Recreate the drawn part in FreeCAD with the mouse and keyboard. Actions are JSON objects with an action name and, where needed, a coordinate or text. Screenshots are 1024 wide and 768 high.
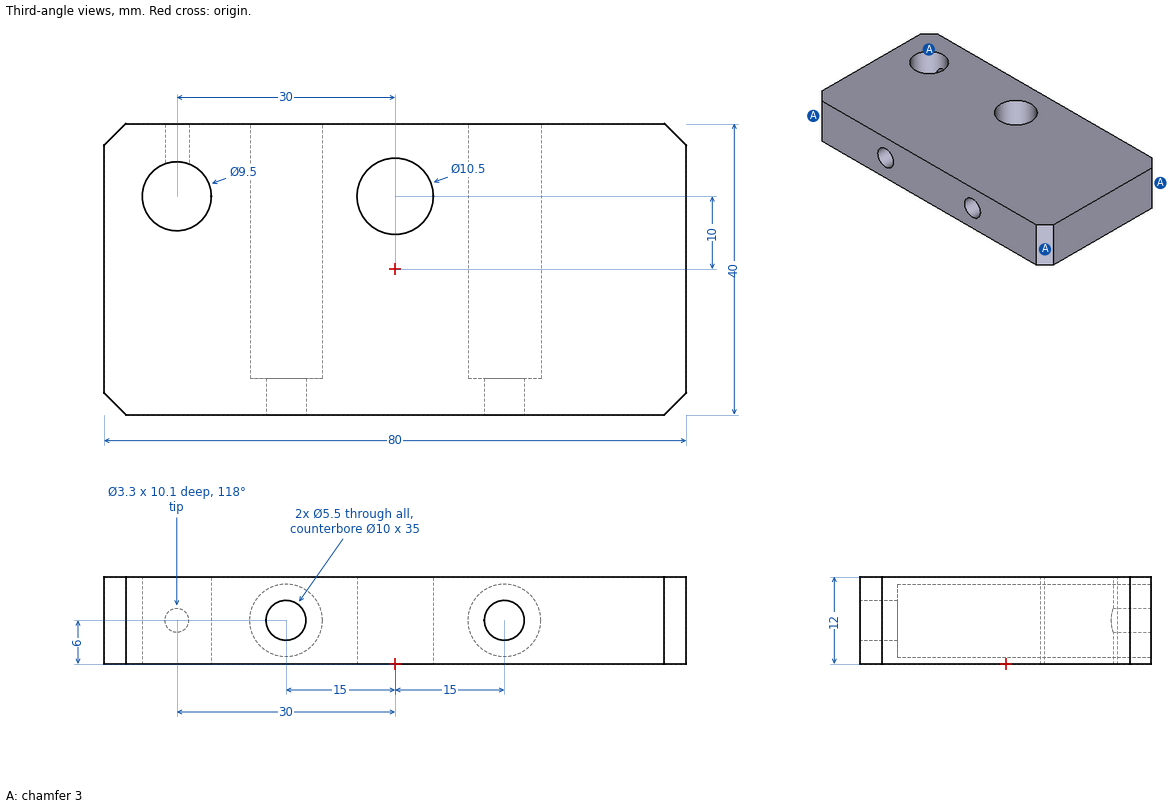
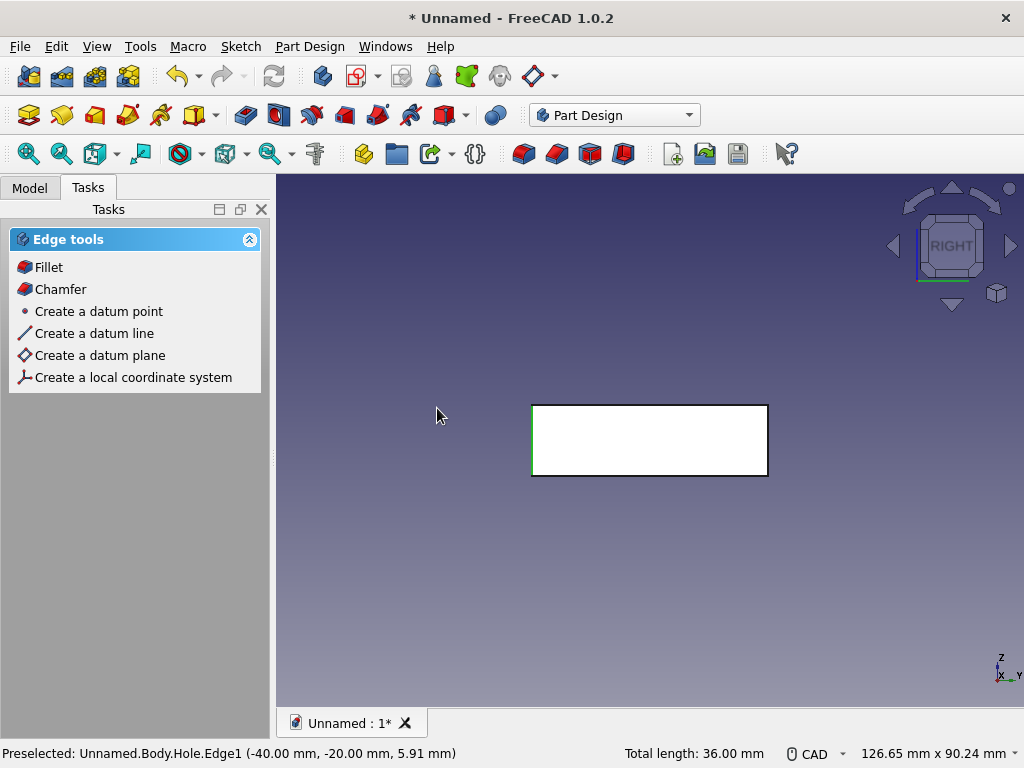
{"action": "left_click", "coordinate": [768, 439], "text": "ctrl"}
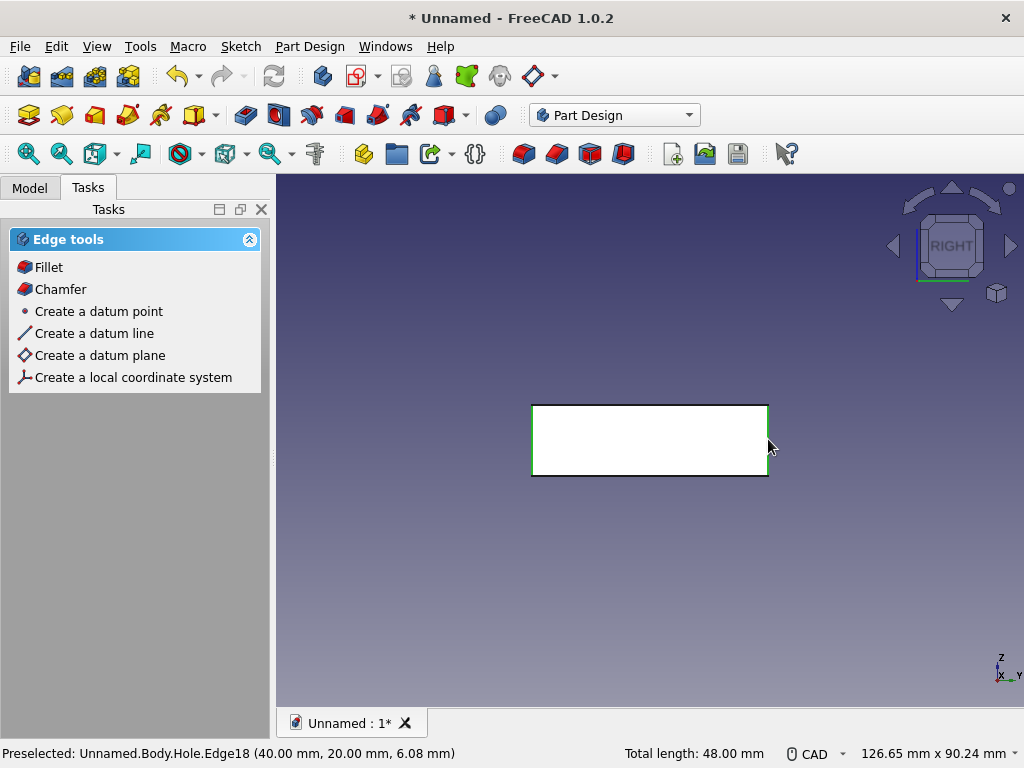
{"action": "left_click", "coordinate": [557, 154]}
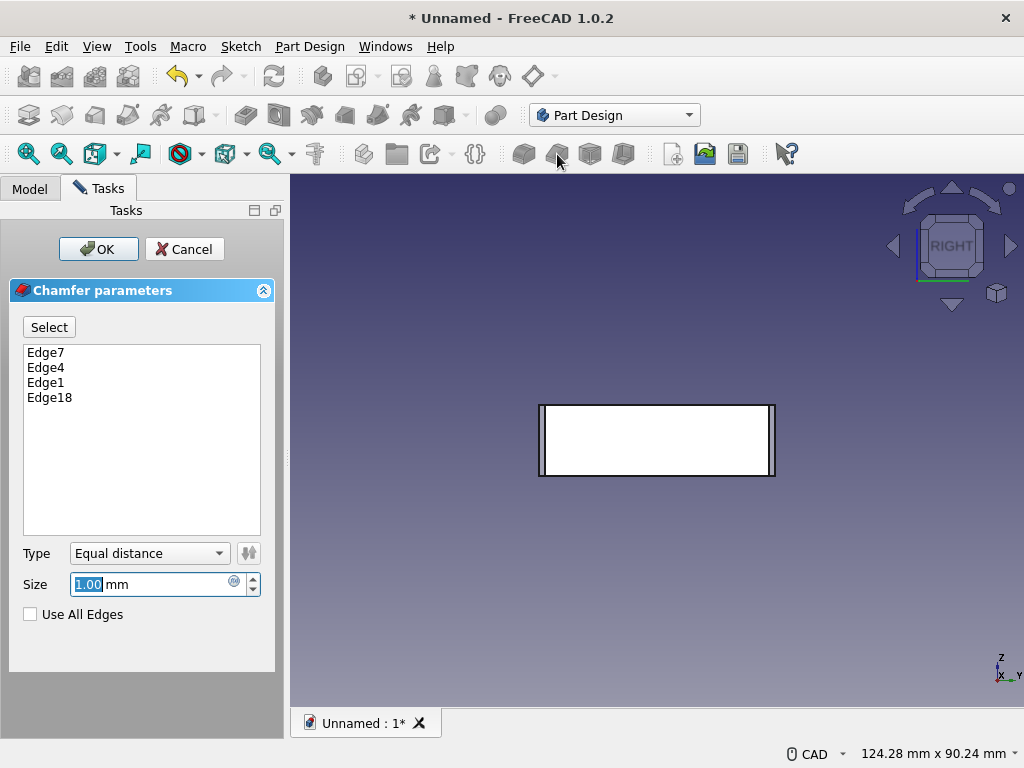
{"action": "type", "text": "3"}
{"action": "key", "text": "Tab"}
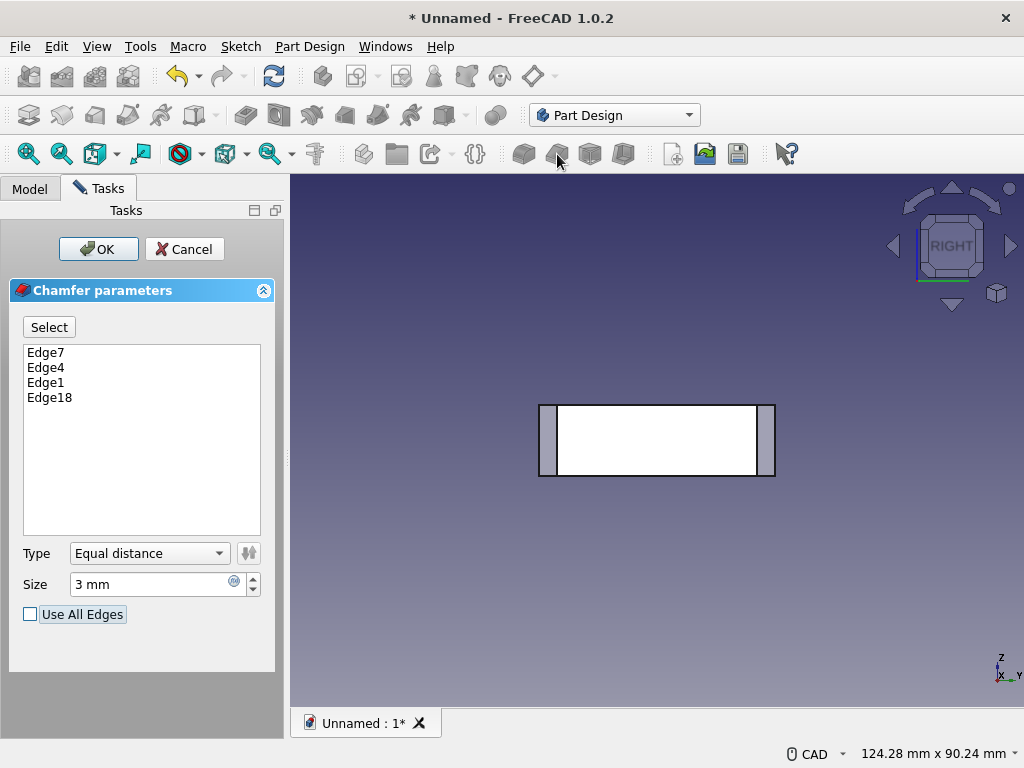
{"action": "left_click", "coordinate": [99, 249]}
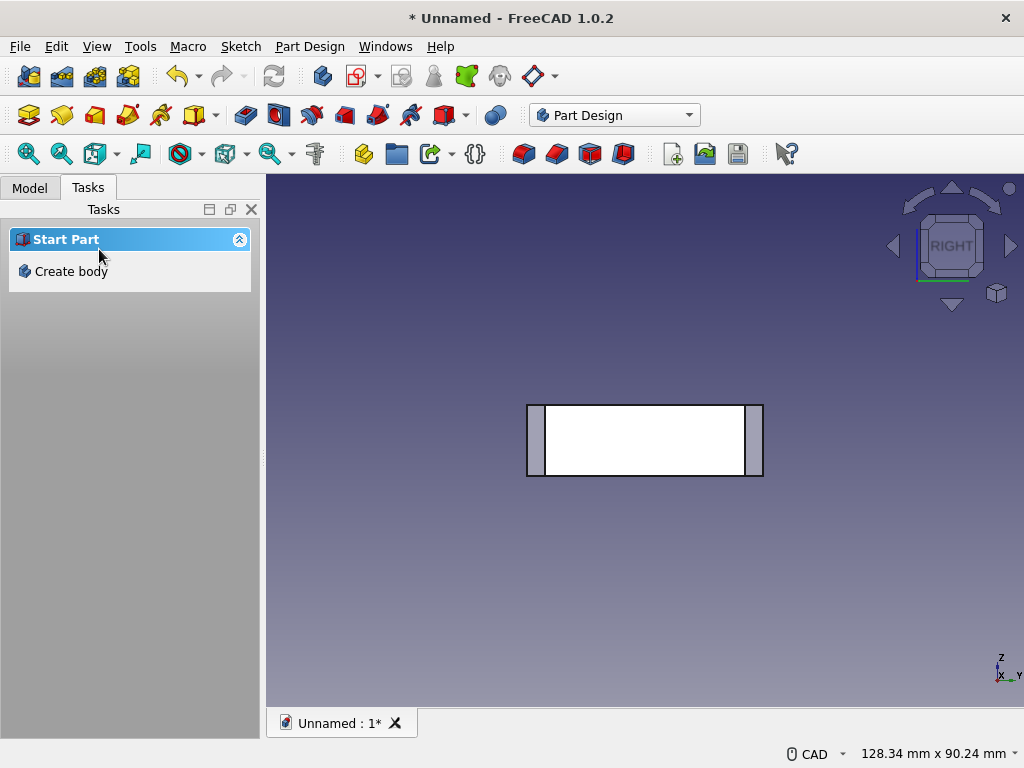
{"action": "left_click", "coordinate": [29, 154]}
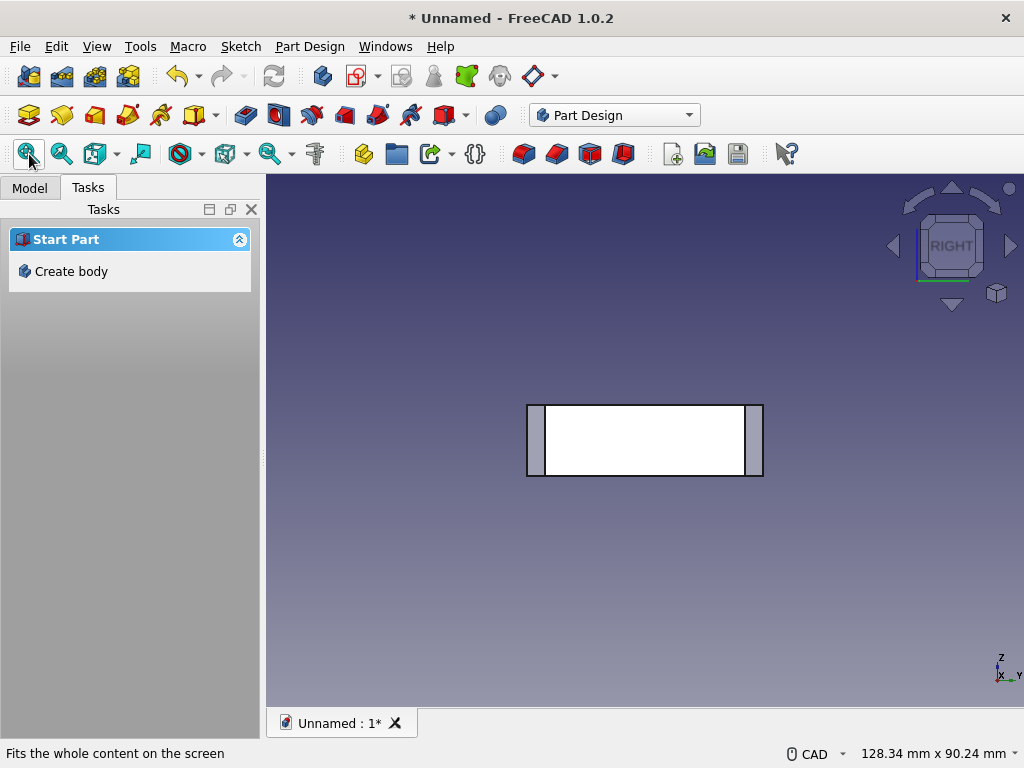
{"action": "key", "text": "4"}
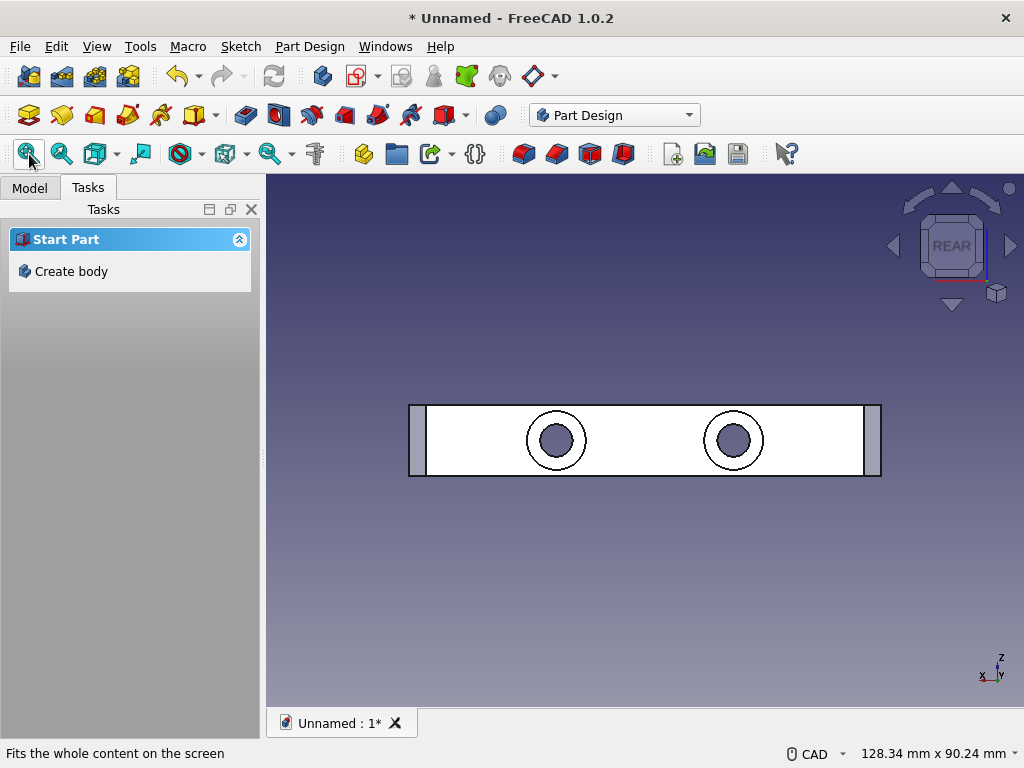
{"action": "left_click", "coordinate": [645, 439]}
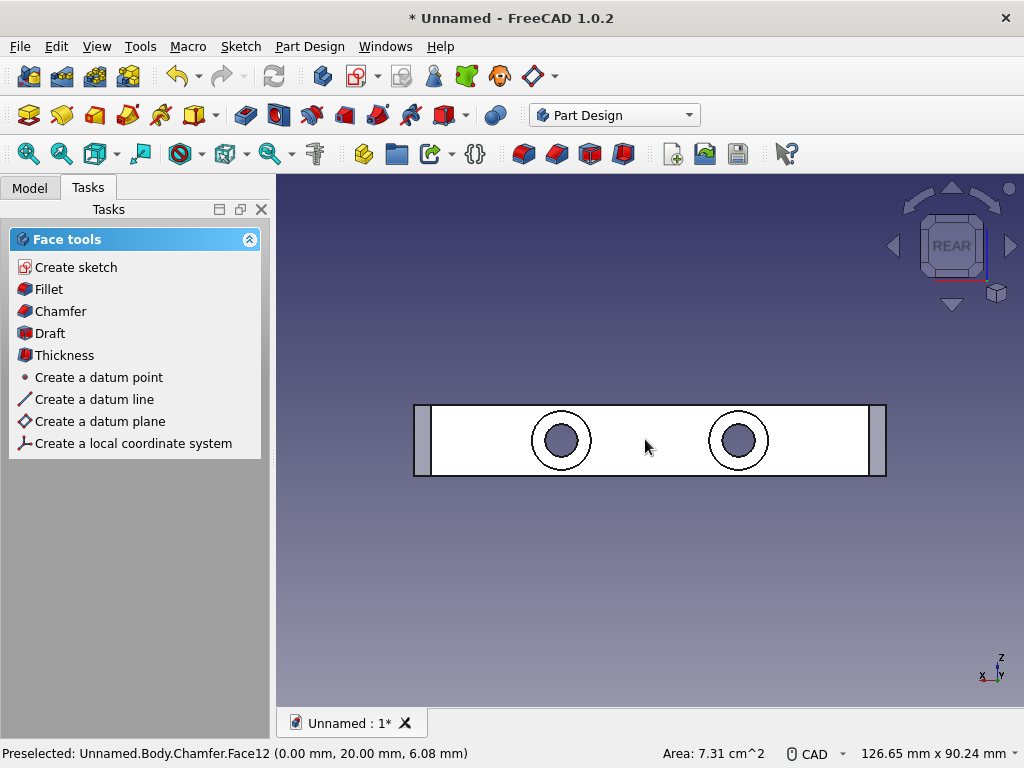
{"action": "left_click", "coordinate": [356, 76]}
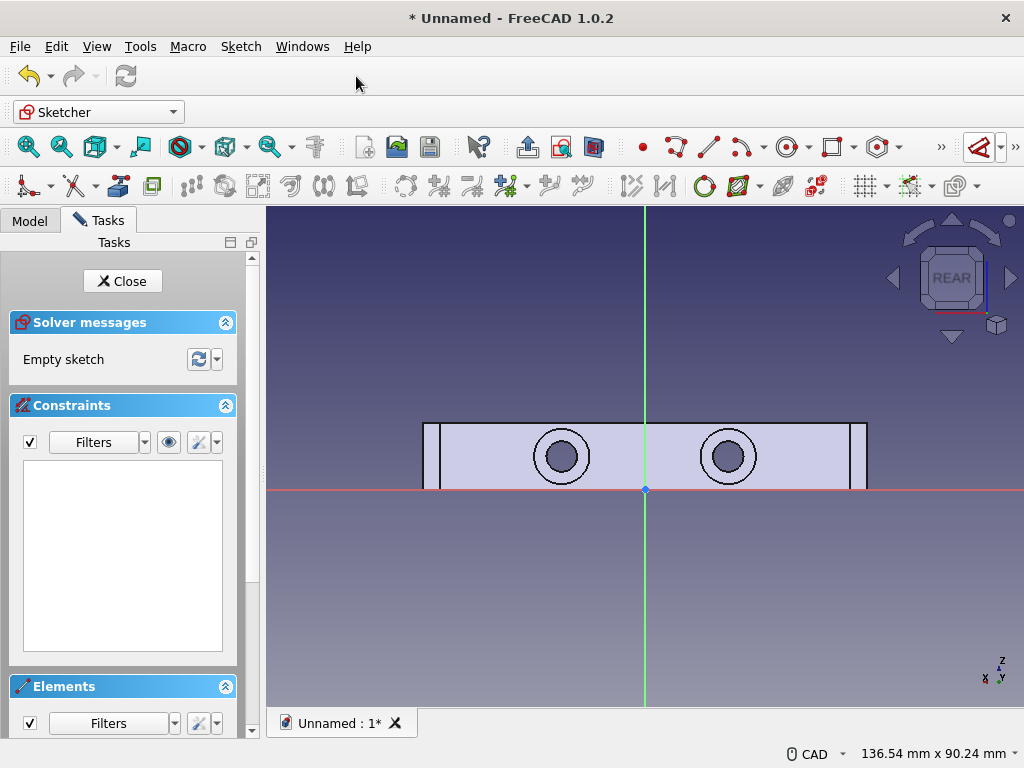
{"action": "scroll", "coordinate": [827, 456], "scroll_direction": "up", "scroll_amount": 14}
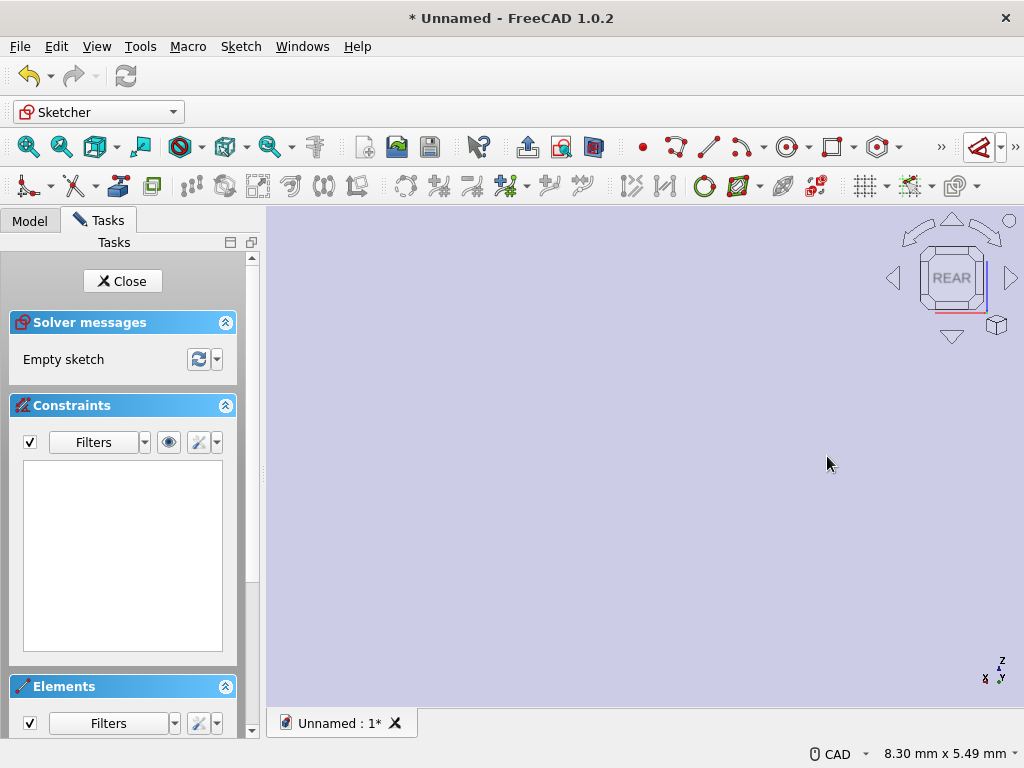
{"action": "left_click", "coordinate": [786, 148]}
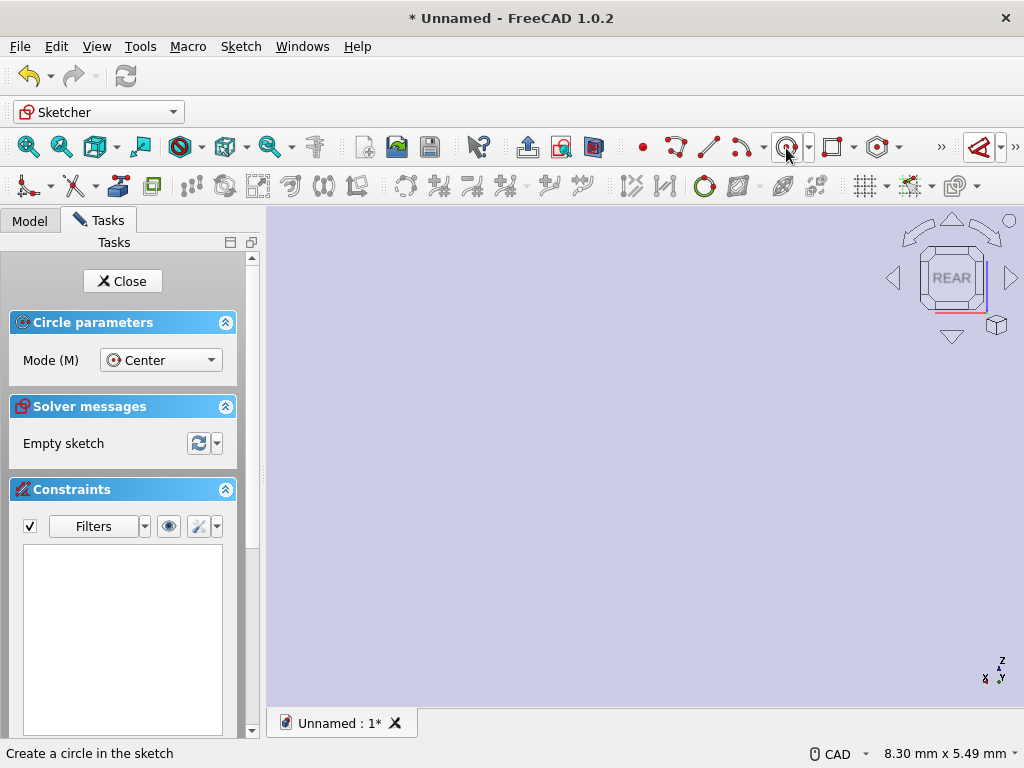
{"action": "left_click", "coordinate": [561, 456]}
{"action": "left_click", "coordinate": [668, 350]}
{"action": "key", "text": "Escape"}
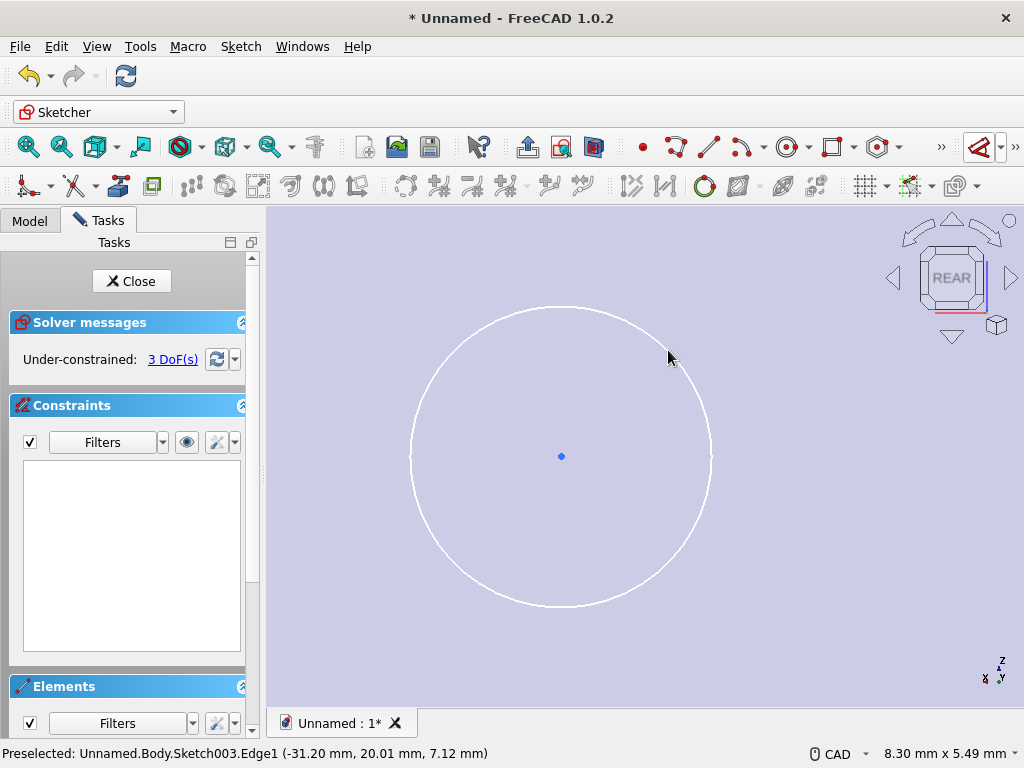
{"action": "left_click", "coordinate": [667, 350]}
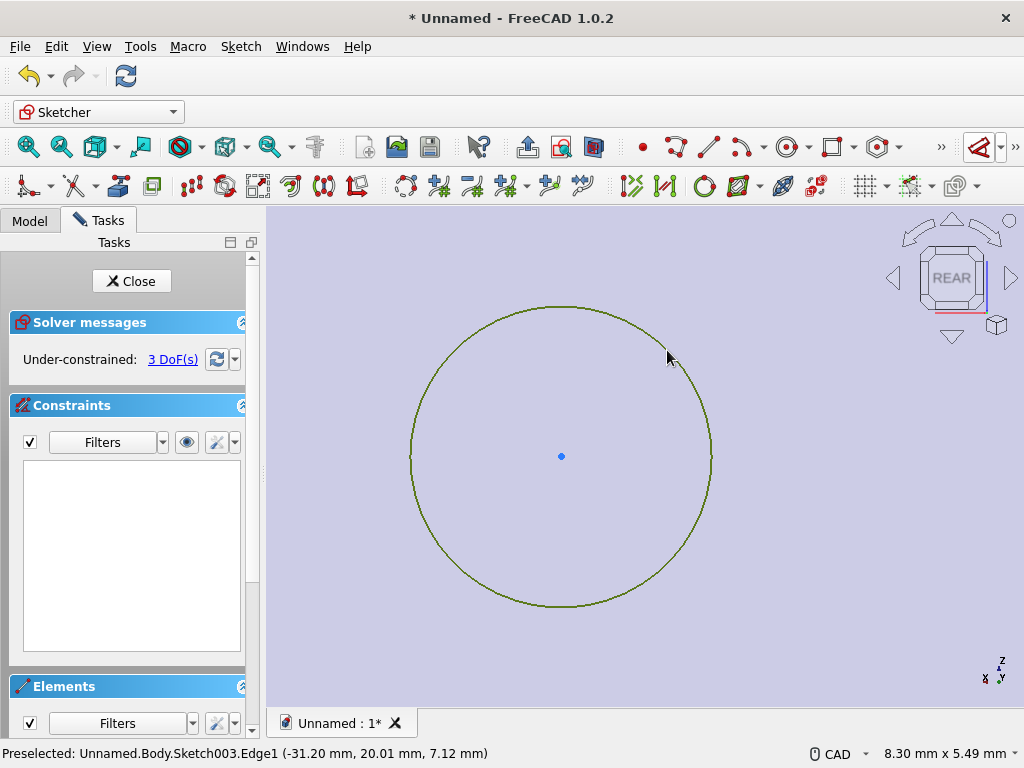
{"action": "key", "text": "k o"}